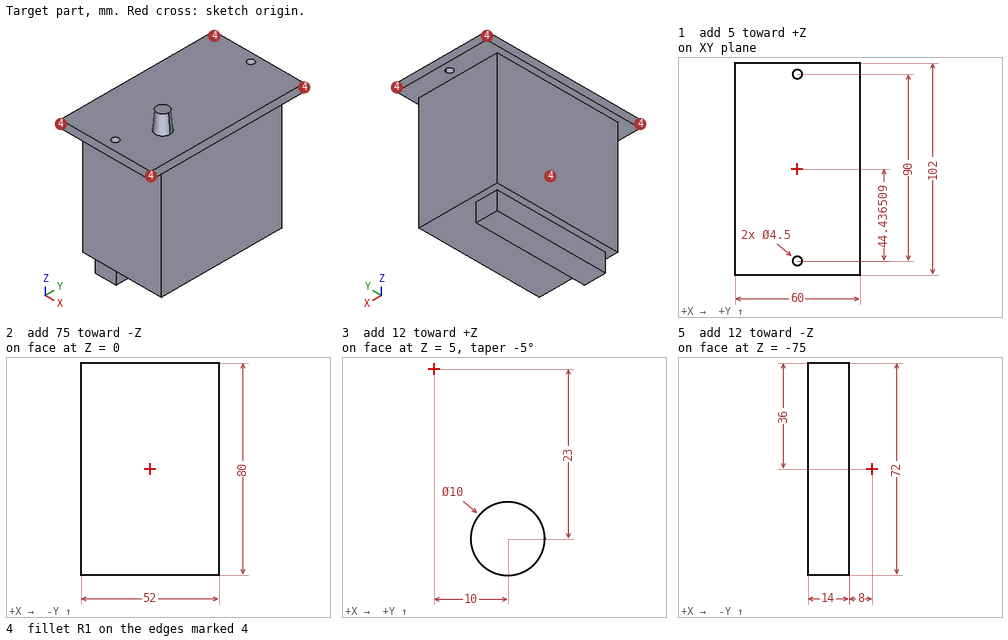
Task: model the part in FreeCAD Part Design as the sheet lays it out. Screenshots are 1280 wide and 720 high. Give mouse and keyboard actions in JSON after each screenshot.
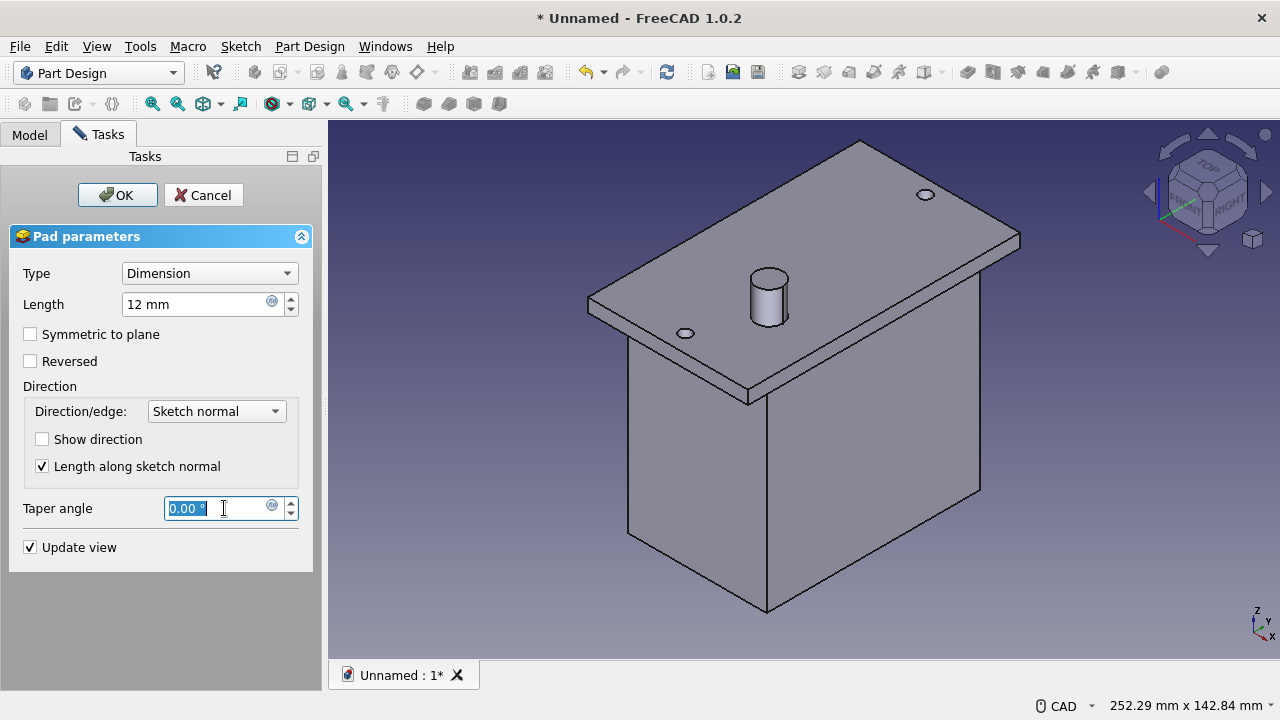
{"action": "type", "text": "-5"}
{"action": "key", "text": "Tab"}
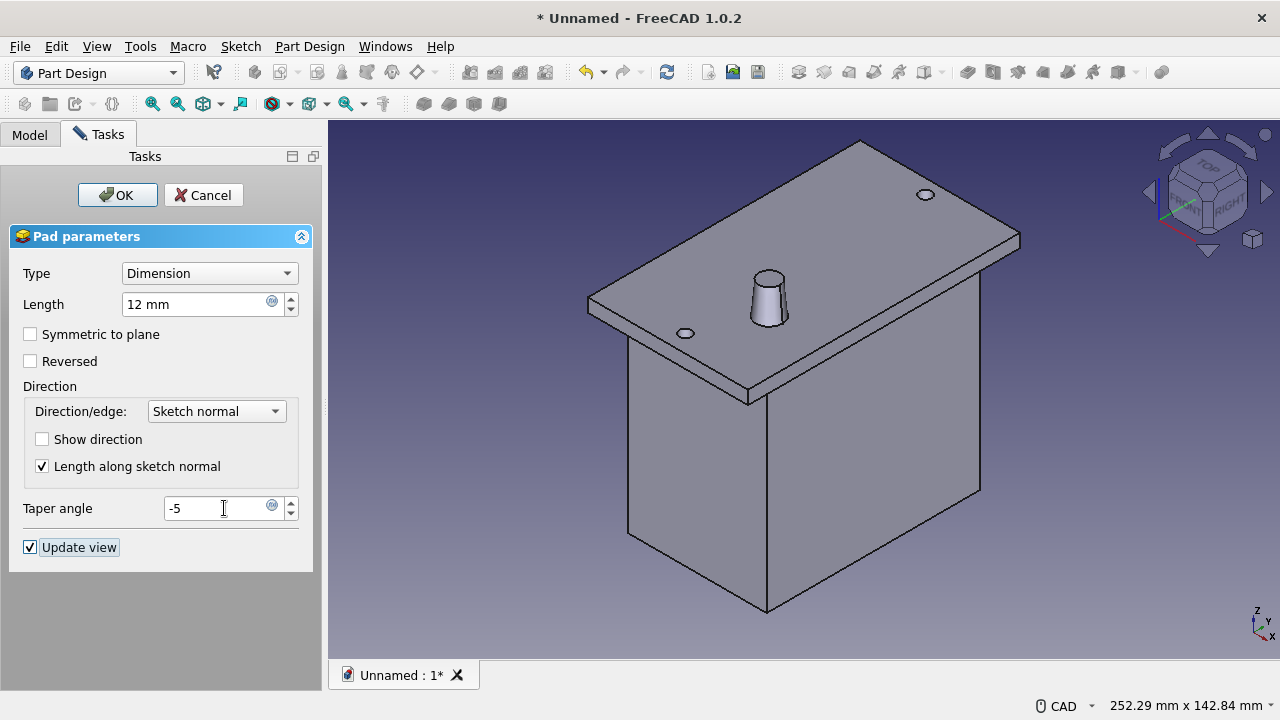
{"action": "left_click", "coordinate": [118, 195]}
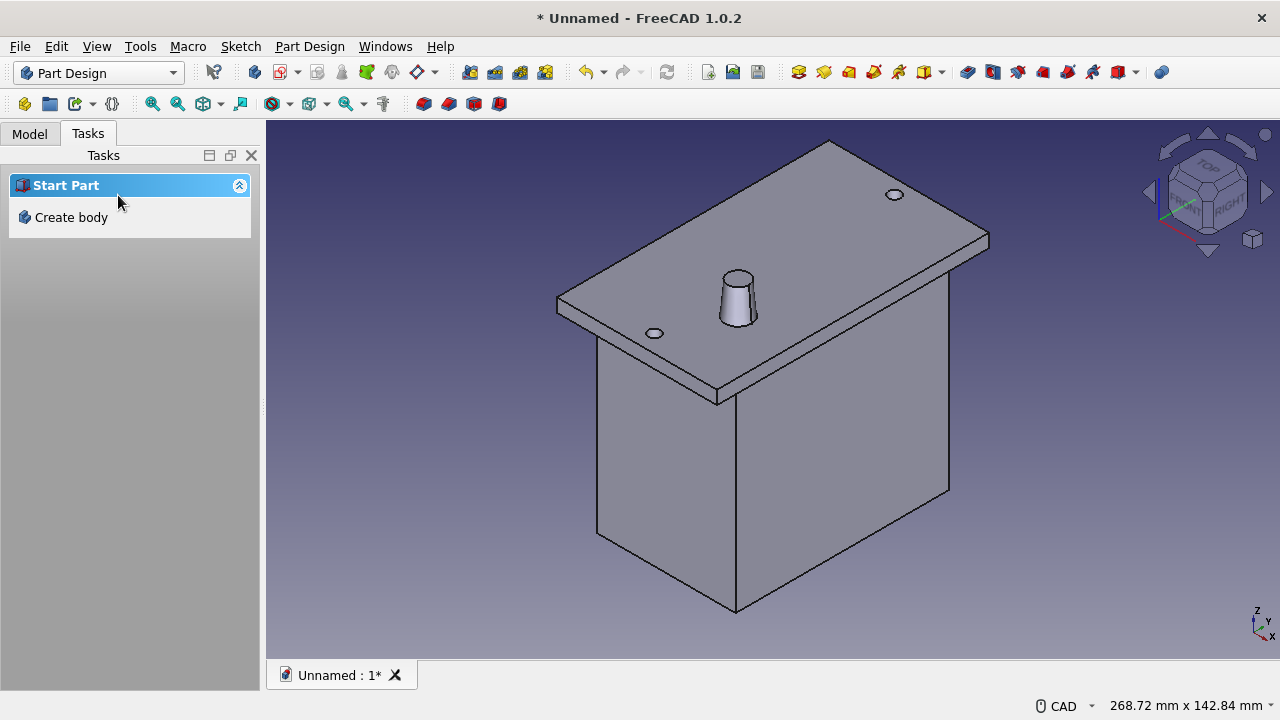
{"action": "left_click", "coordinate": [153, 104]}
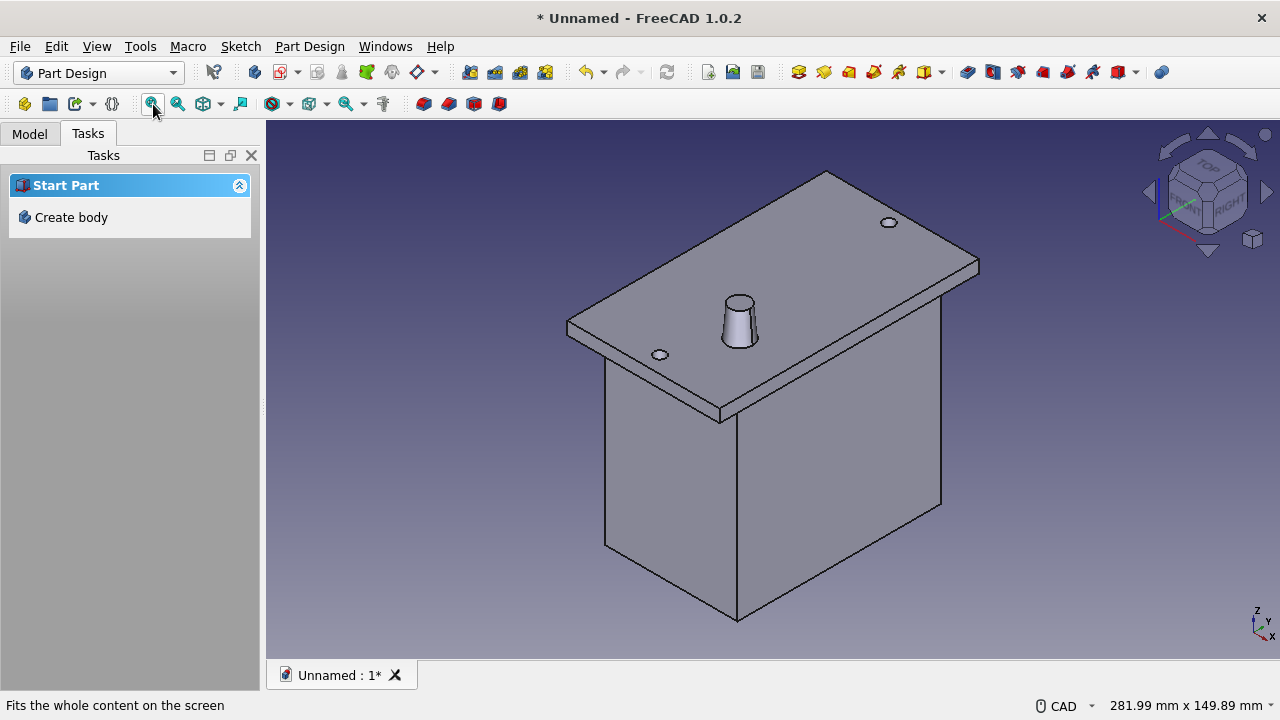
{"action": "left_click", "coordinate": [720, 415]}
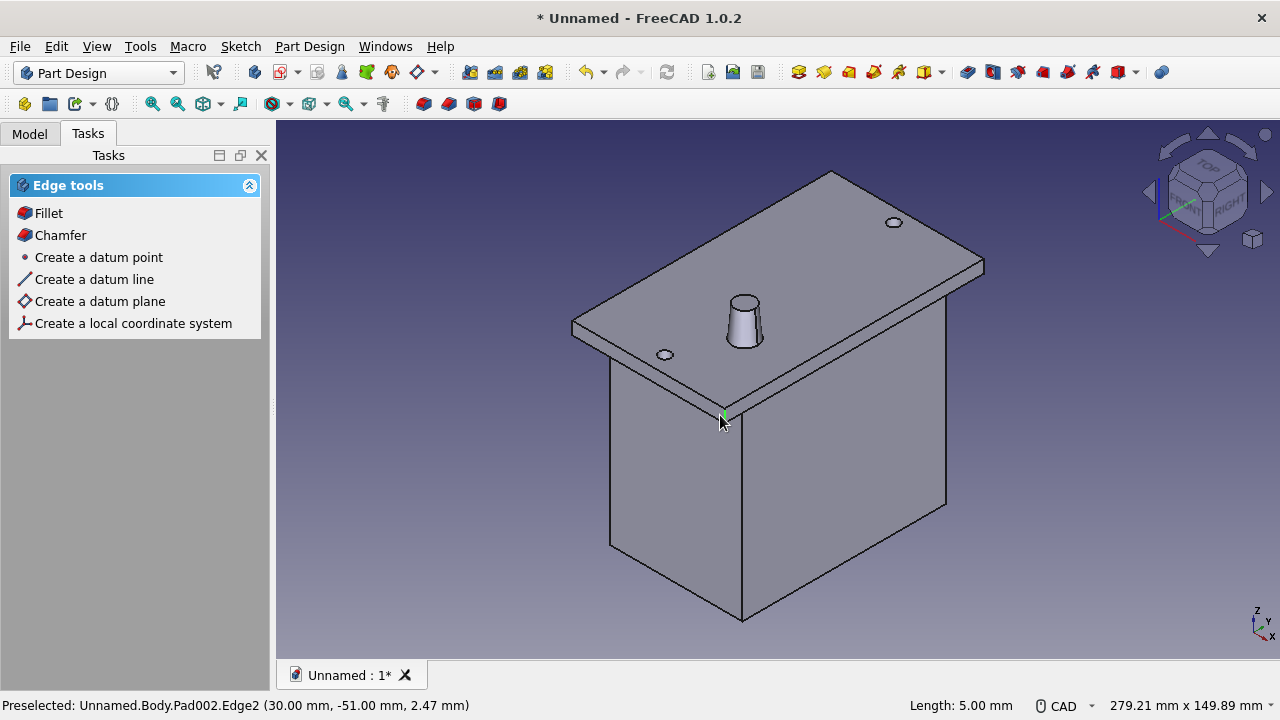
{"action": "scroll", "coordinate": [572, 327], "scroll_direction": "up", "scroll_amount": 4}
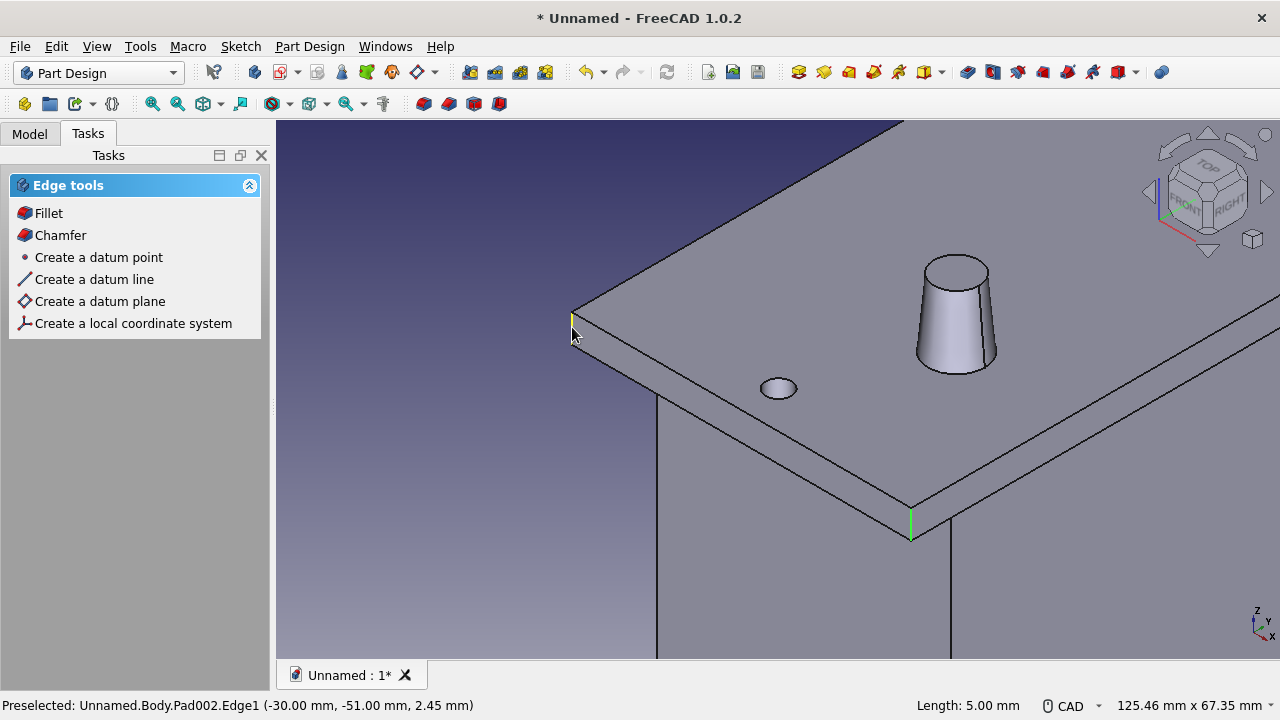
{"action": "key", "text": "v f"}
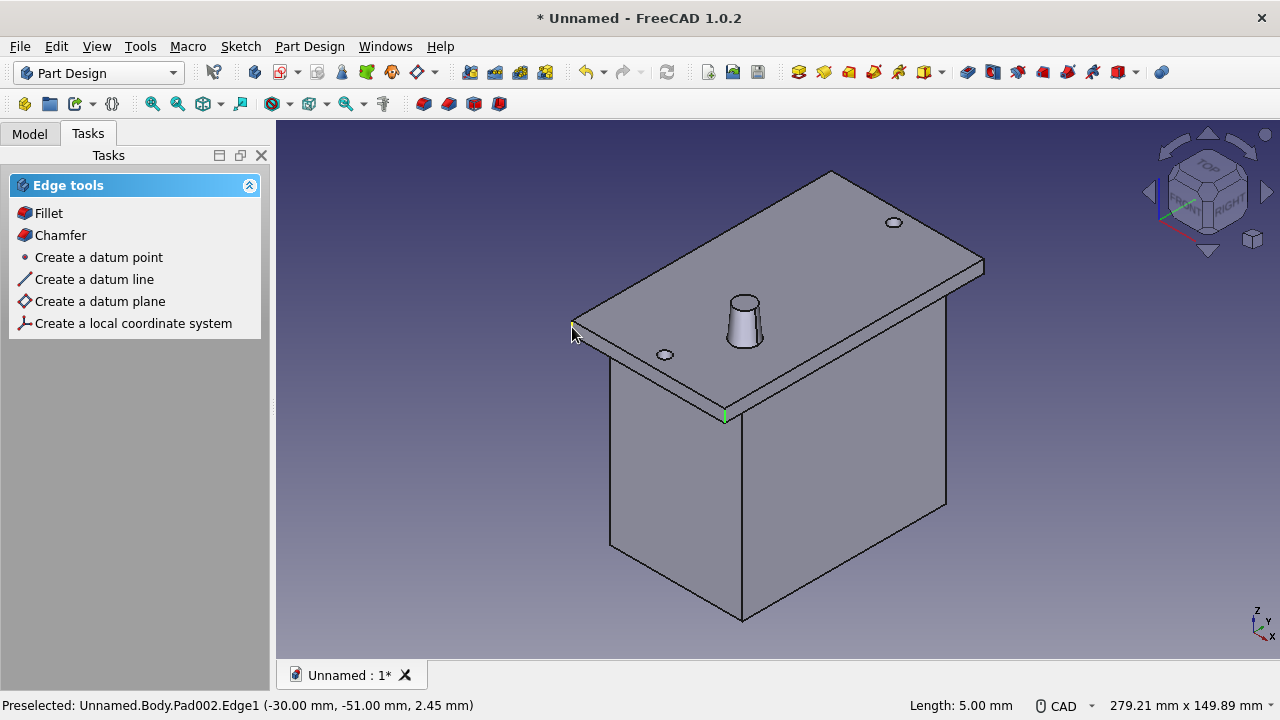
{"action": "key", "text": "2"}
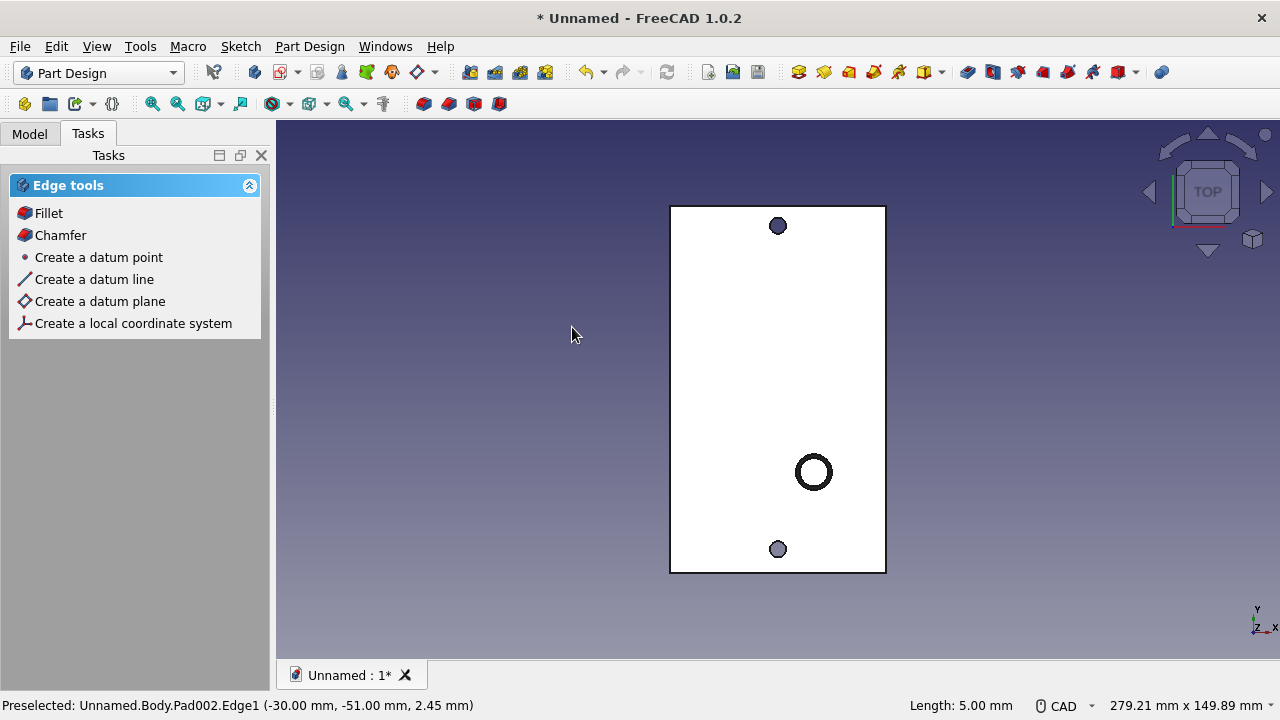
{"action": "scroll", "coordinate": [670, 572], "scroll_direction": "up", "scroll_amount": 4}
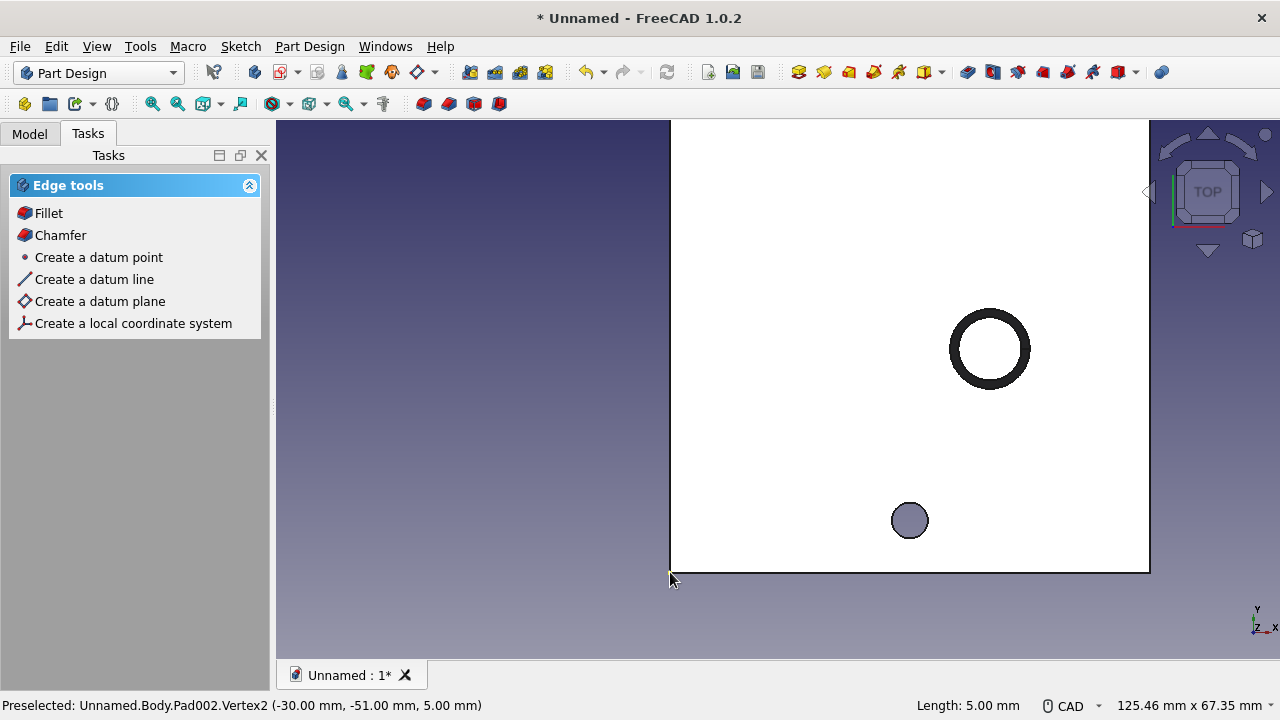
{"action": "left_click", "coordinate": [153, 104]}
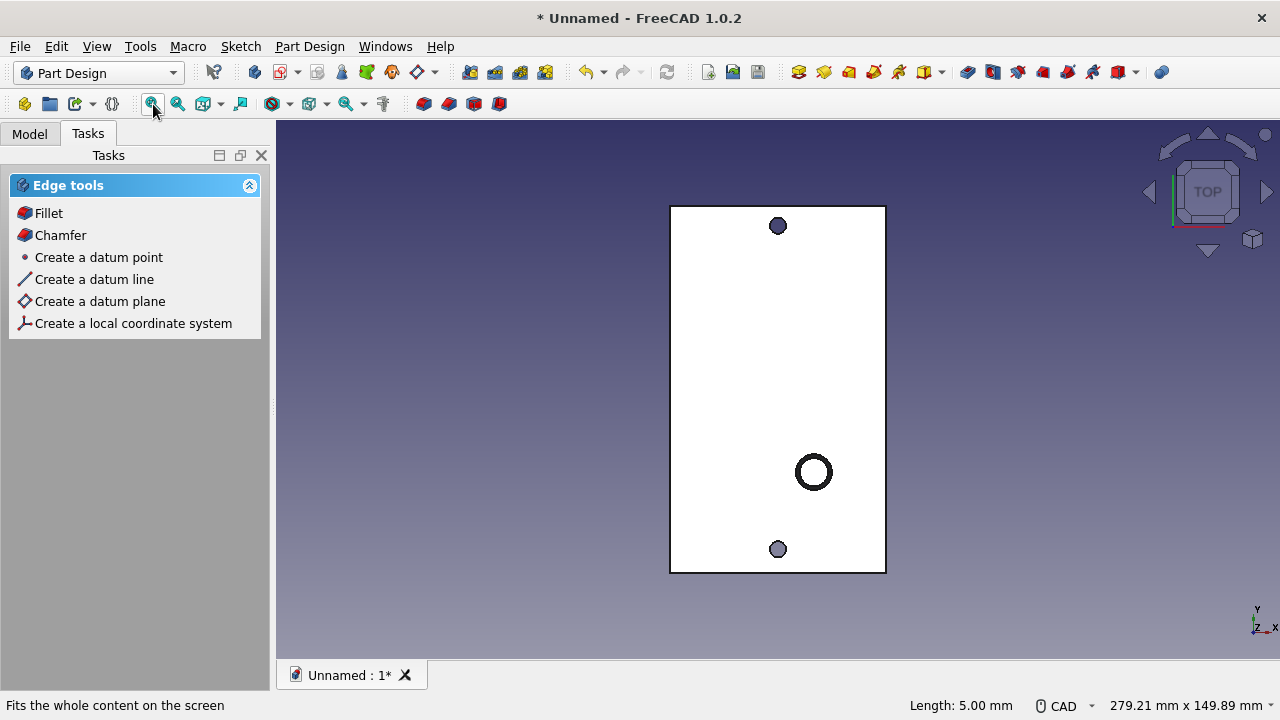
{"action": "key", "text": "0"}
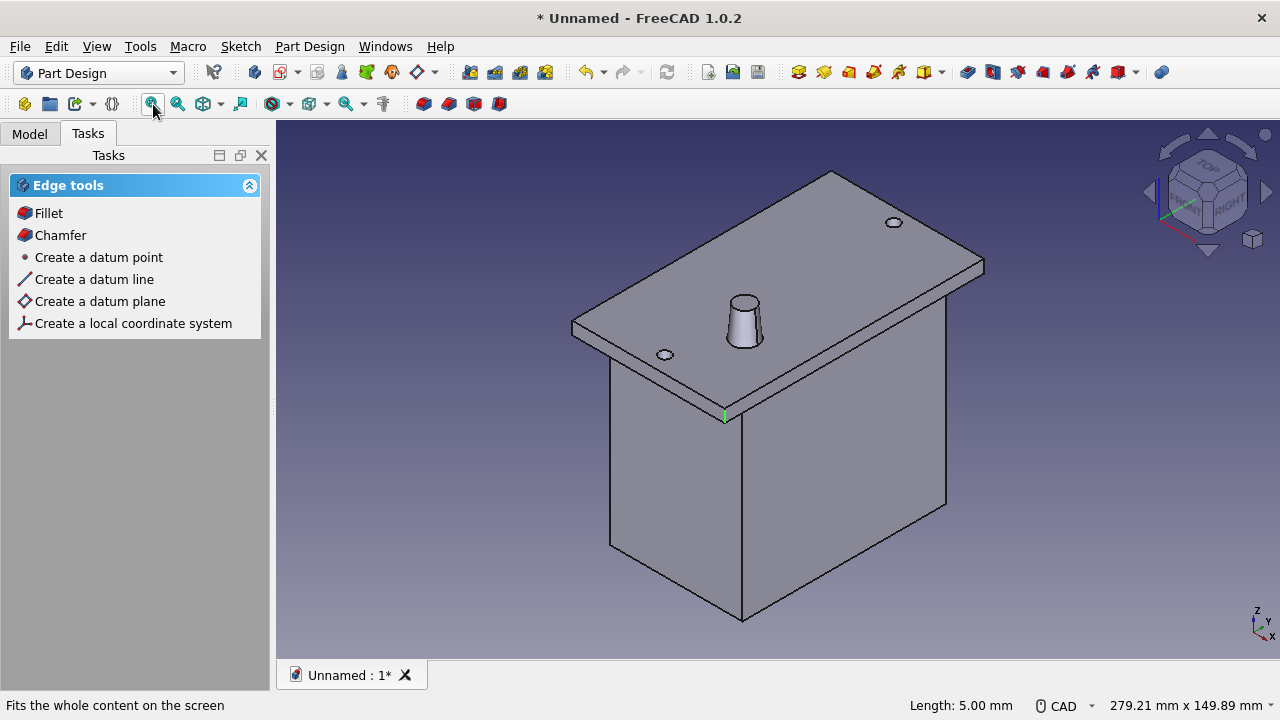
{"action": "scroll", "coordinate": [572, 327], "scroll_direction": "up", "scroll_amount": 4}